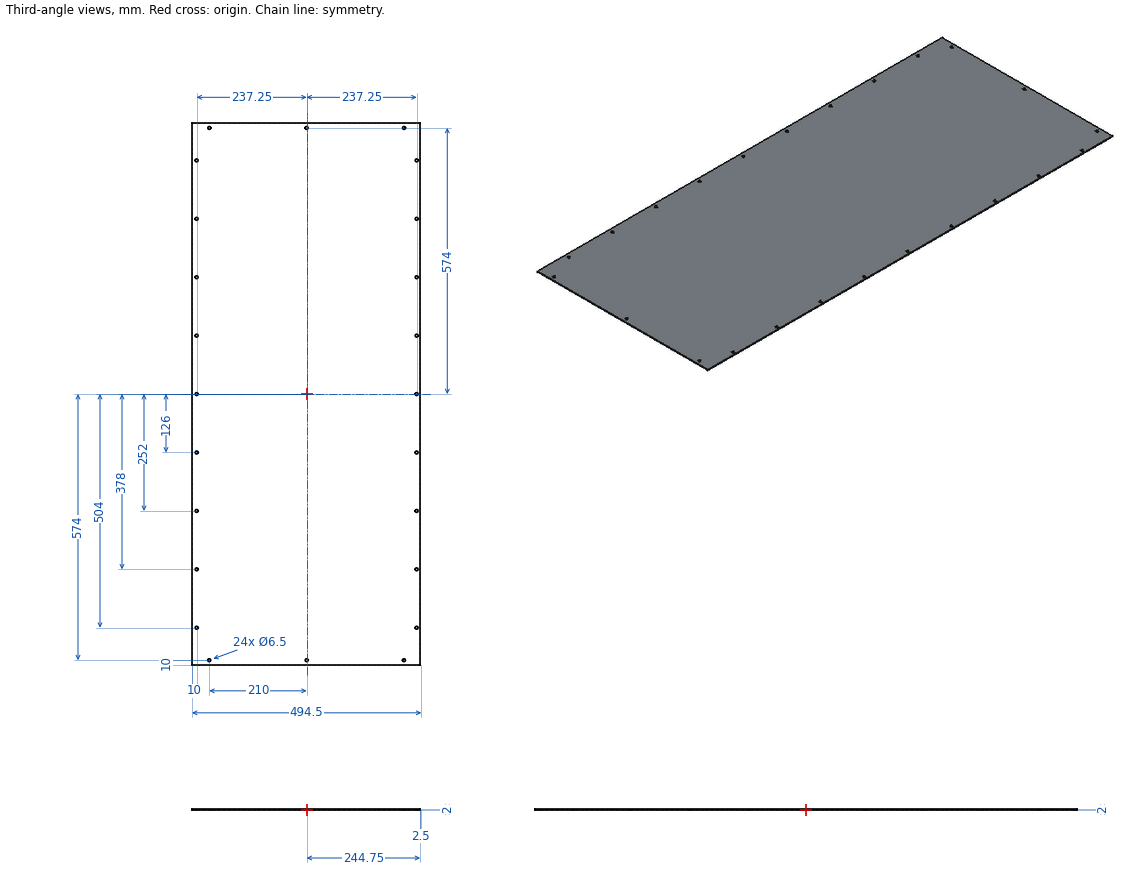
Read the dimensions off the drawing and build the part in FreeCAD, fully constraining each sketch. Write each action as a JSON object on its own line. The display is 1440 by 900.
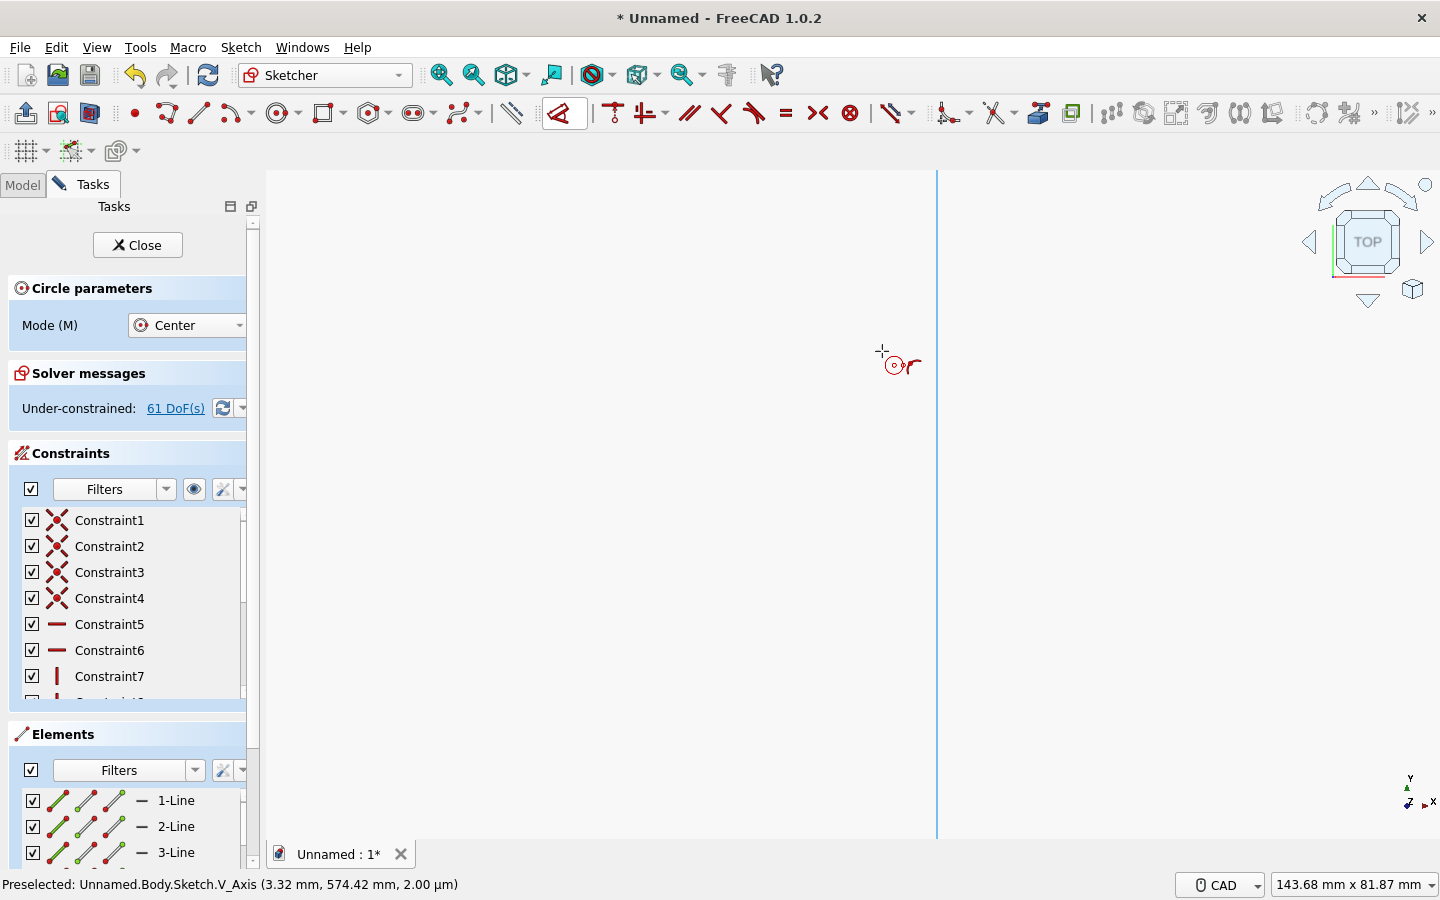
{"action": "scroll", "coordinate": [882, 351], "scroll_direction": "down", "scroll_amount": 15}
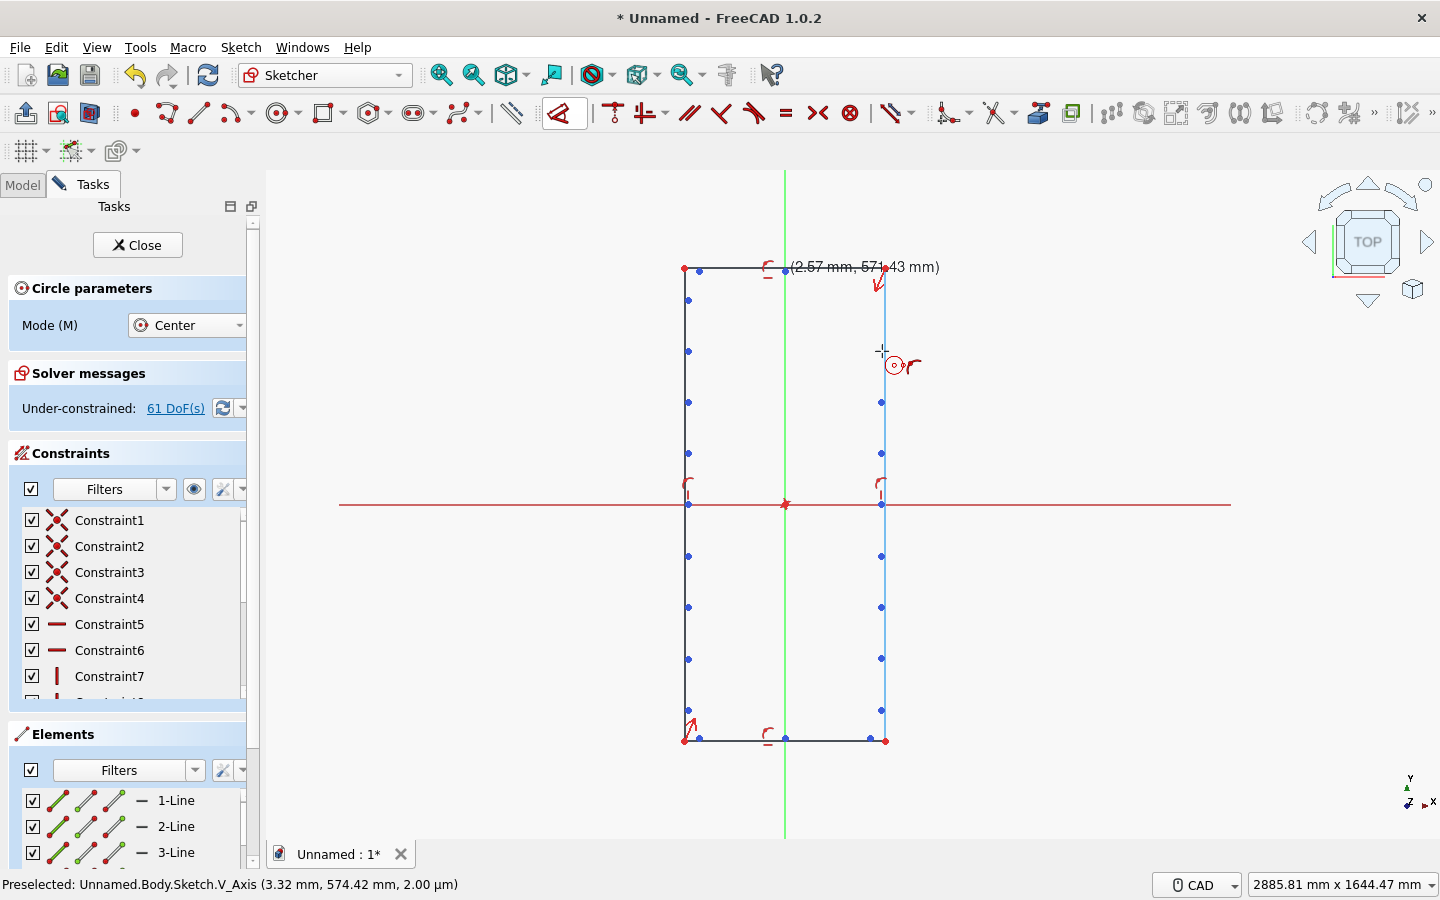
{"action": "scroll", "coordinate": [882, 351], "scroll_direction": "up", "scroll_amount": 7}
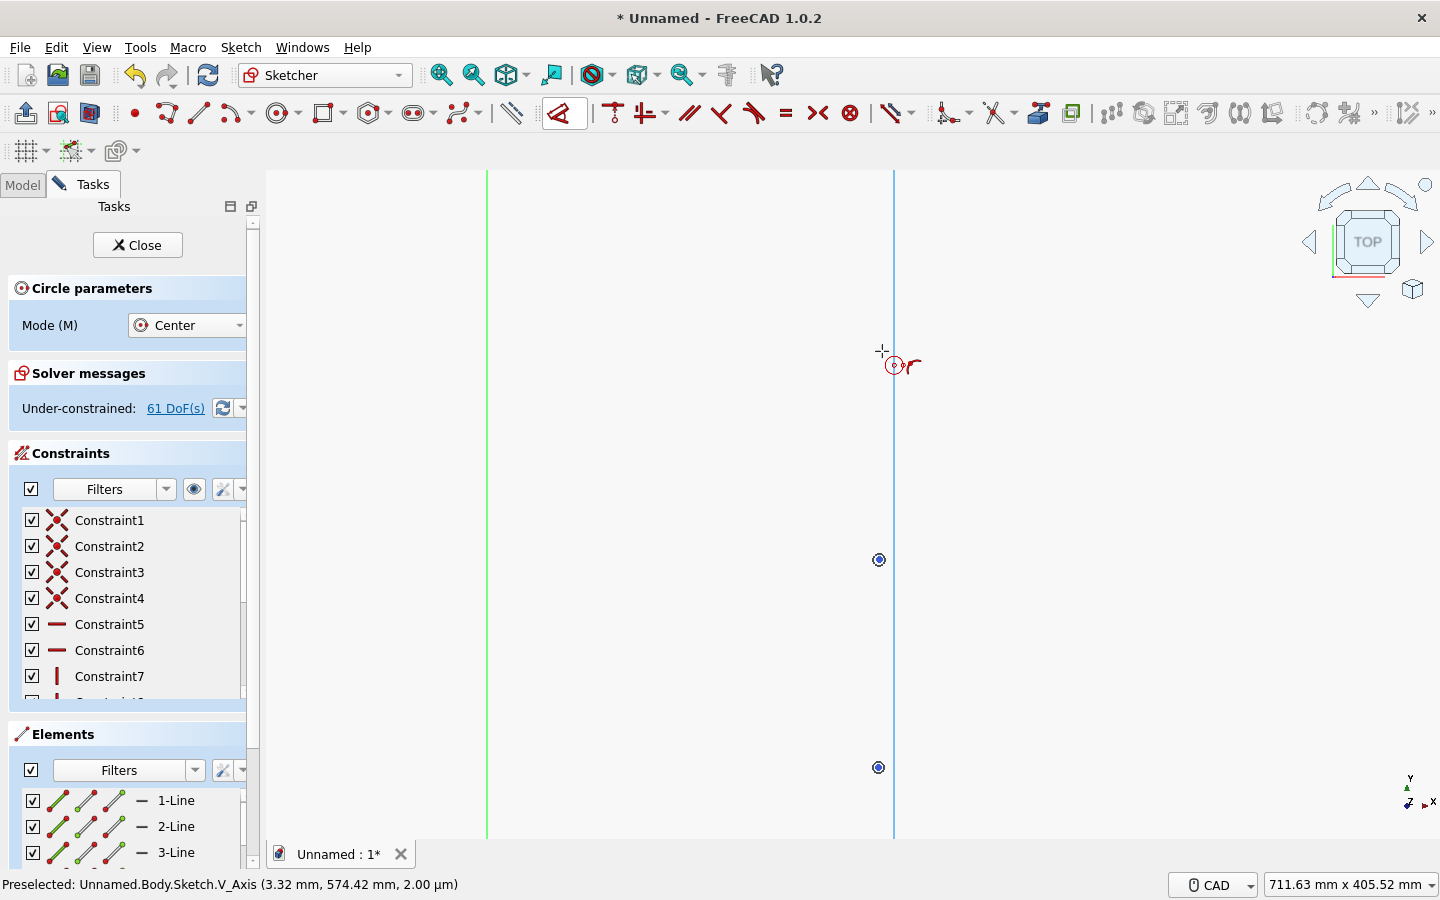
{"action": "left_click", "coordinate": [879, 351]}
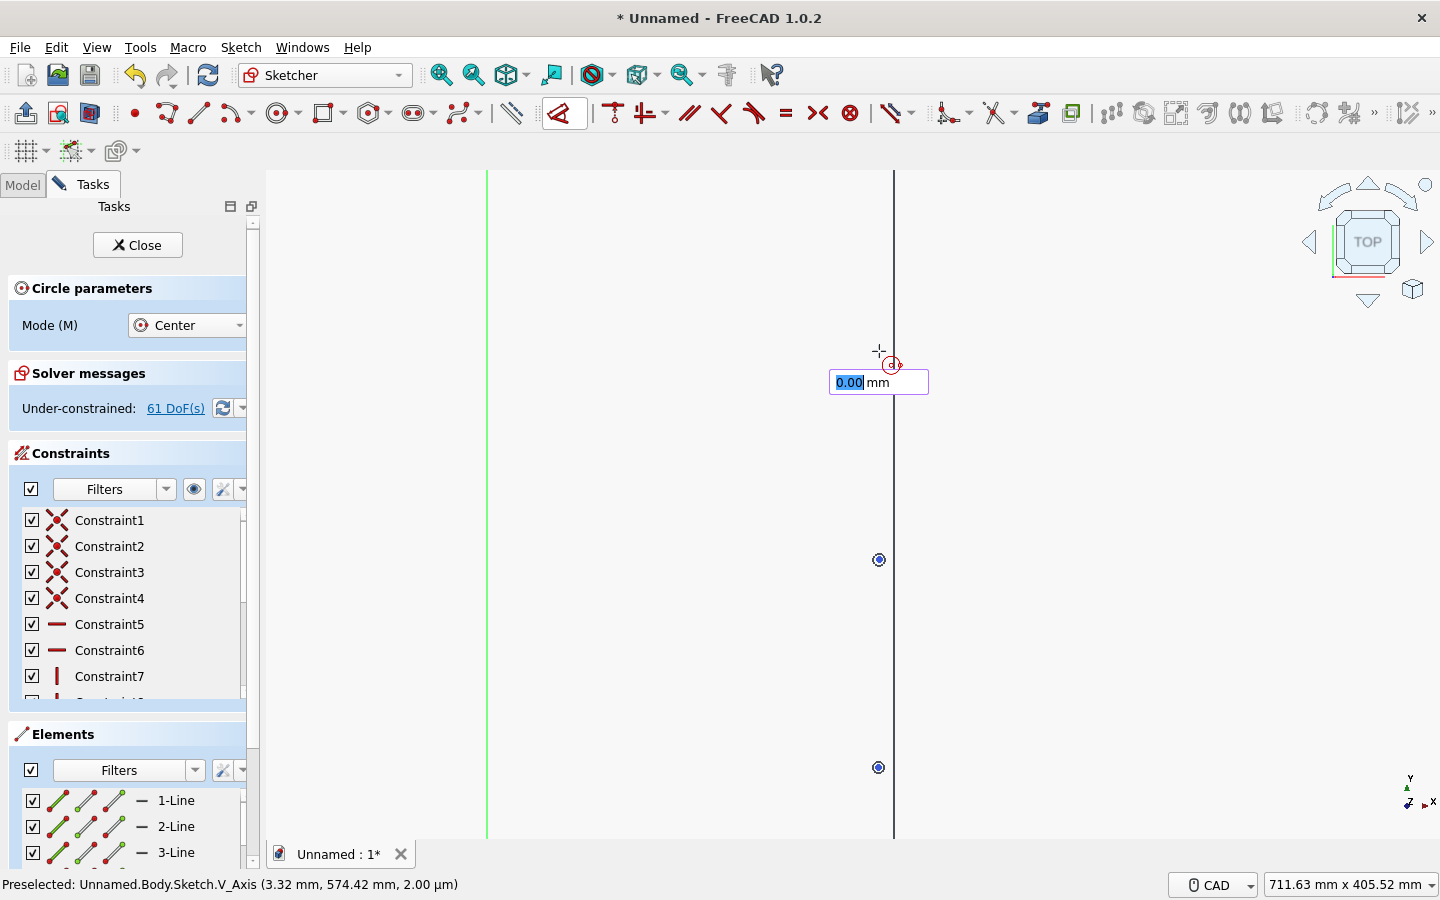
{"action": "scroll", "coordinate": [875, 347], "scroll_direction": "up", "scroll_amount": 6}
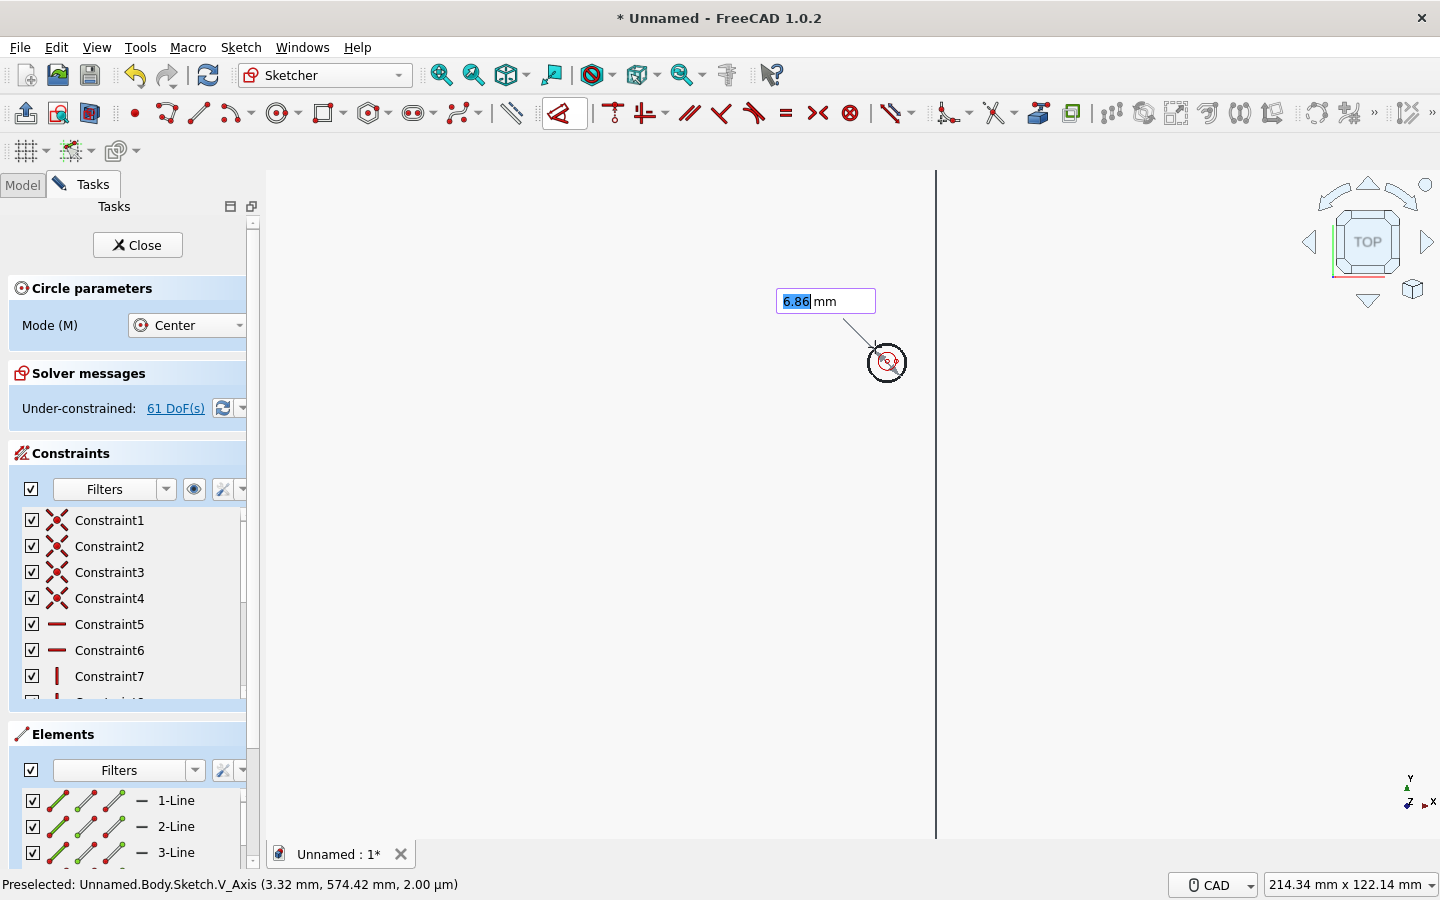
{"action": "left_click", "coordinate": [874, 347]}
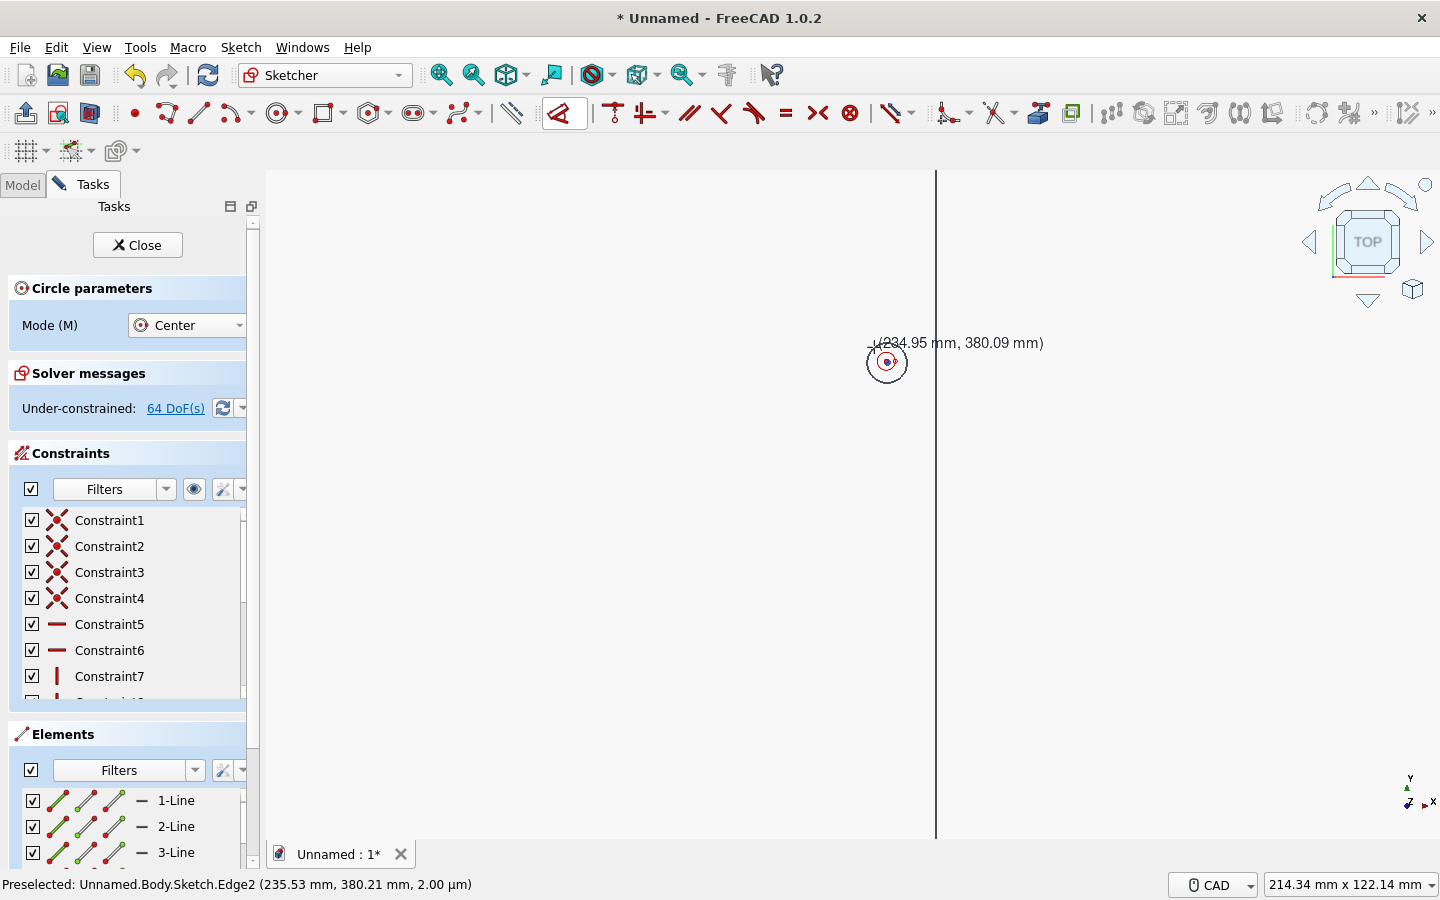
{"action": "scroll", "coordinate": [881, 350], "scroll_direction": "down", "scroll_amount": 13}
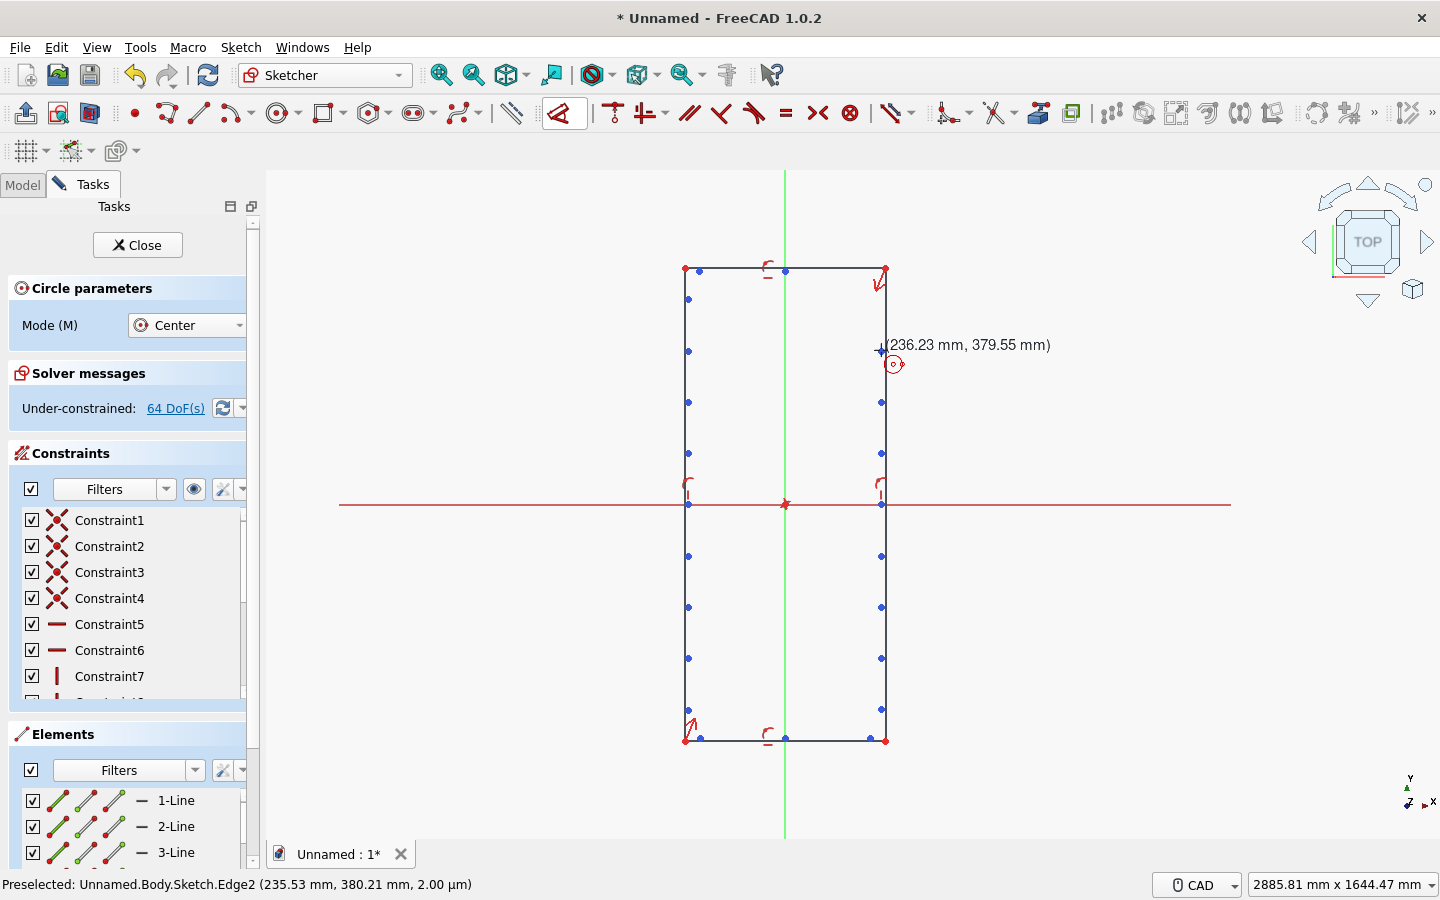
{"action": "scroll", "coordinate": [882, 300], "scroll_direction": "up", "scroll_amount": 15}